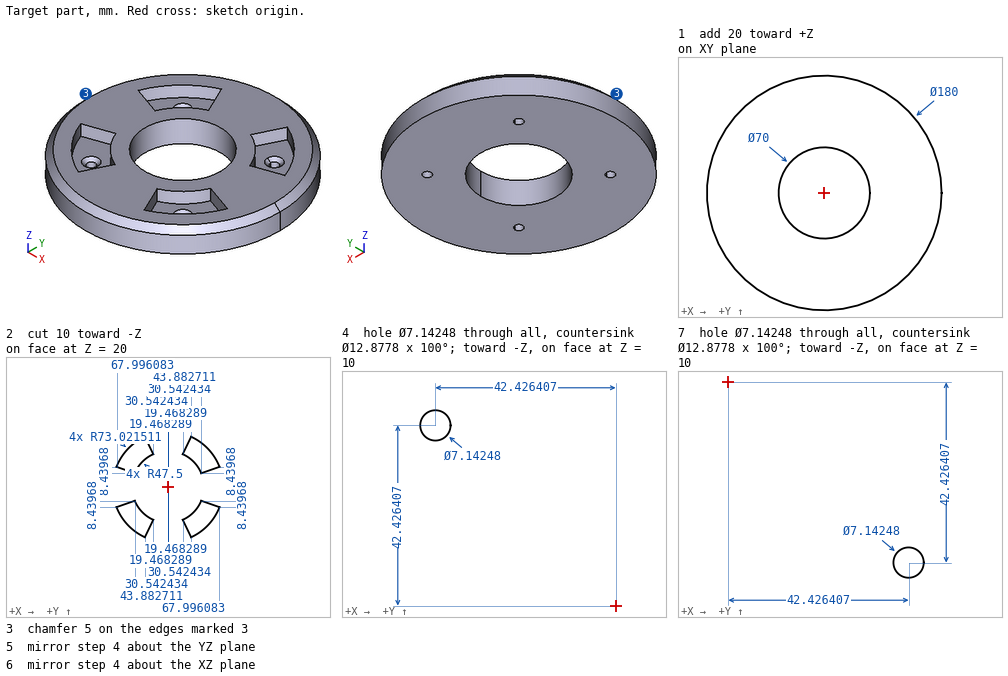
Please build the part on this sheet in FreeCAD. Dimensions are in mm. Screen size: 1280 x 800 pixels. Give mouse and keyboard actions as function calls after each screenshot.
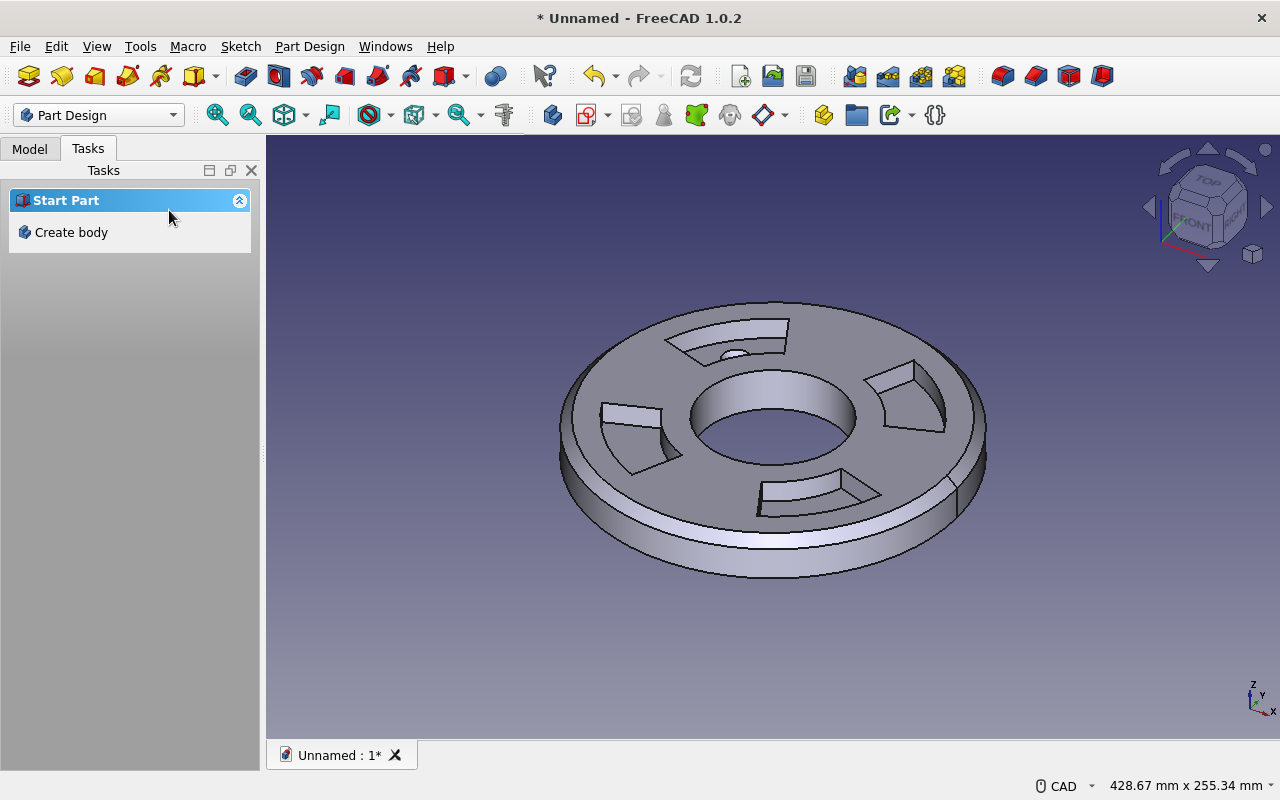
click(30, 148)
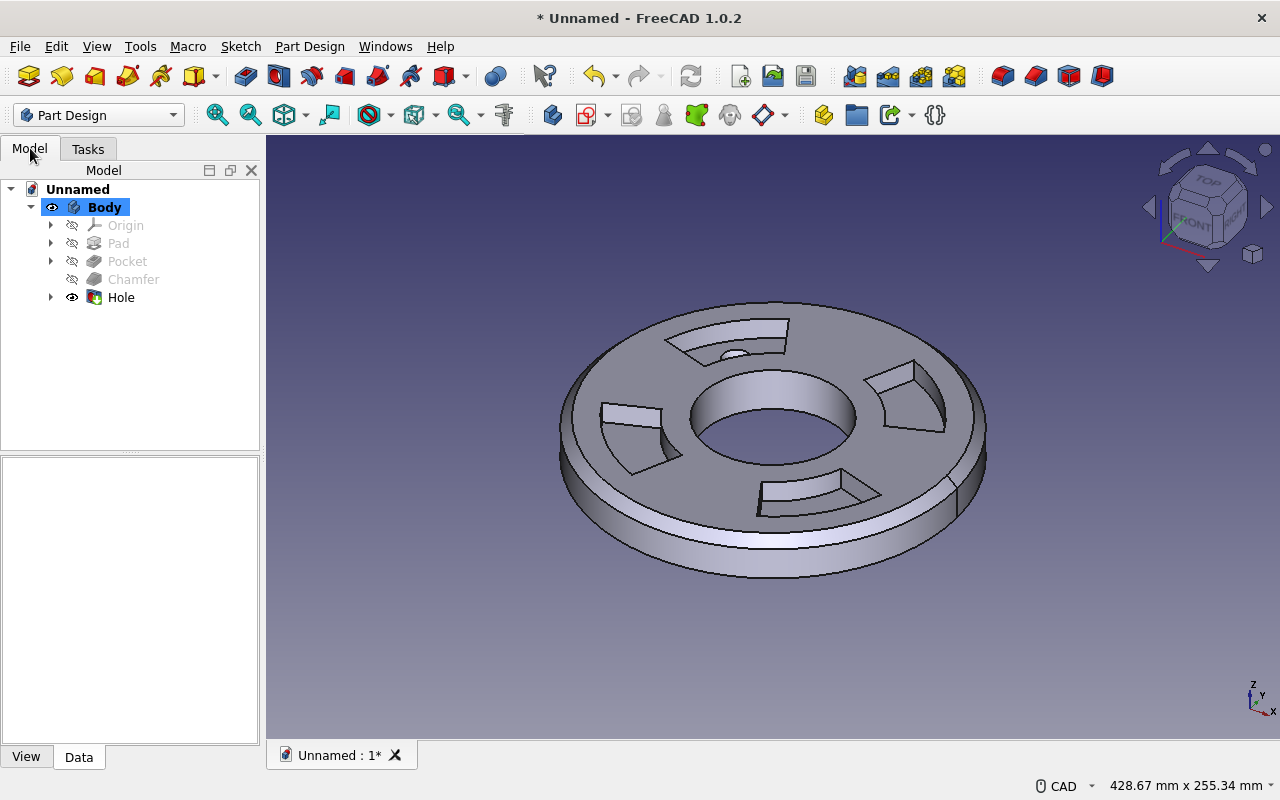
click(117, 297)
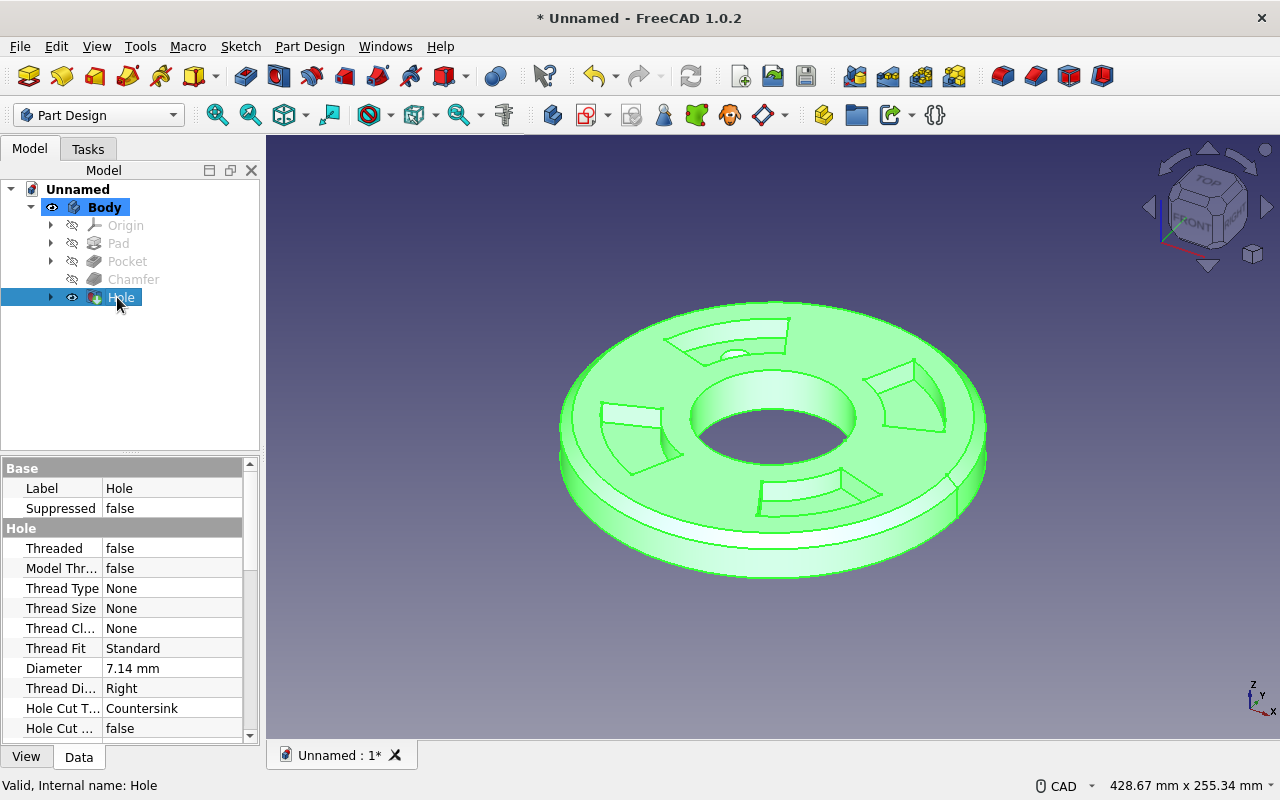
click(855, 76)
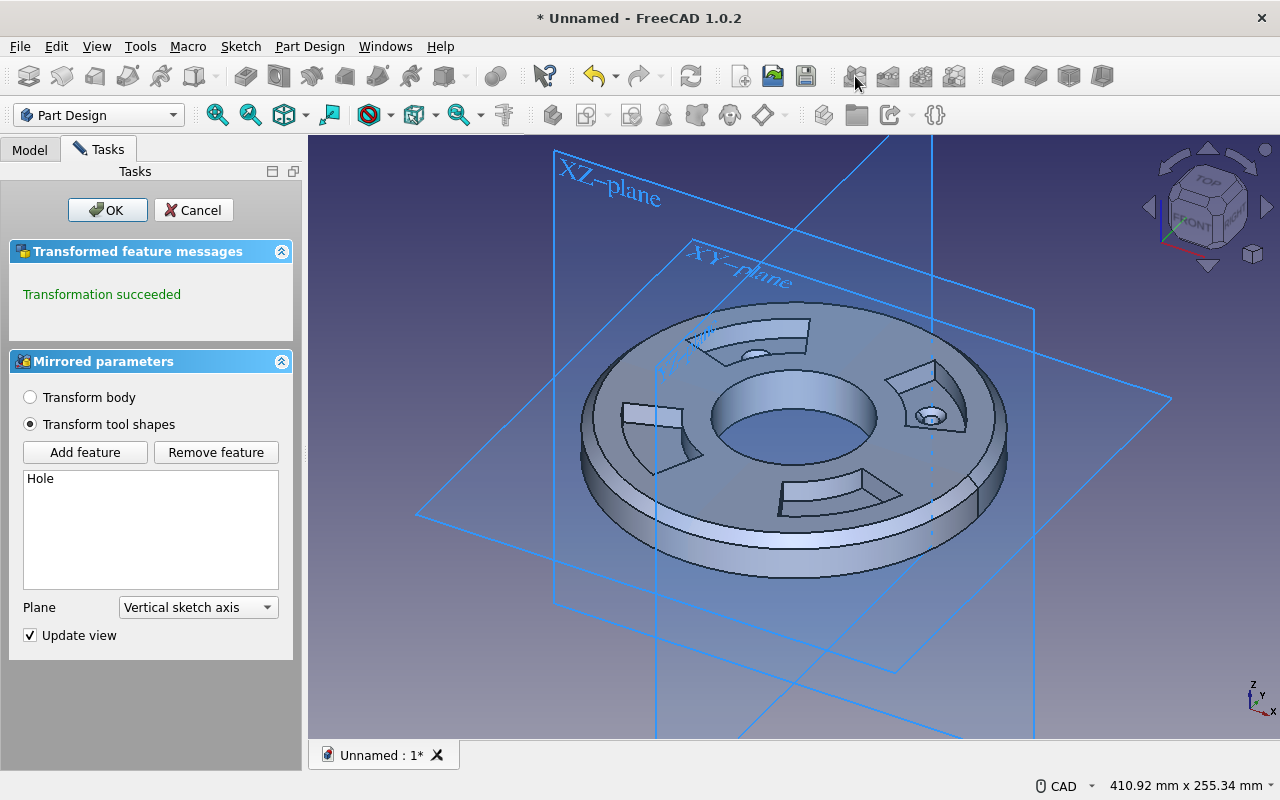
click(199, 608)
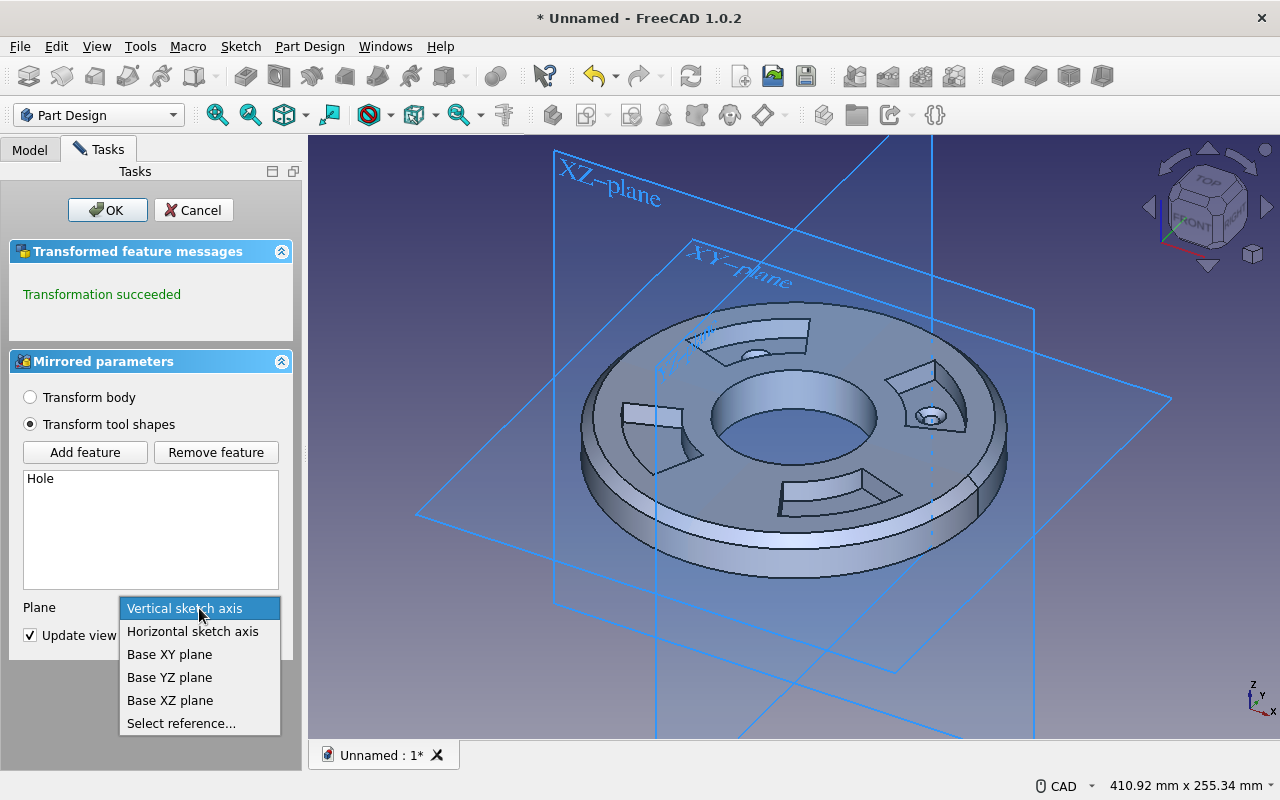
click(198, 678)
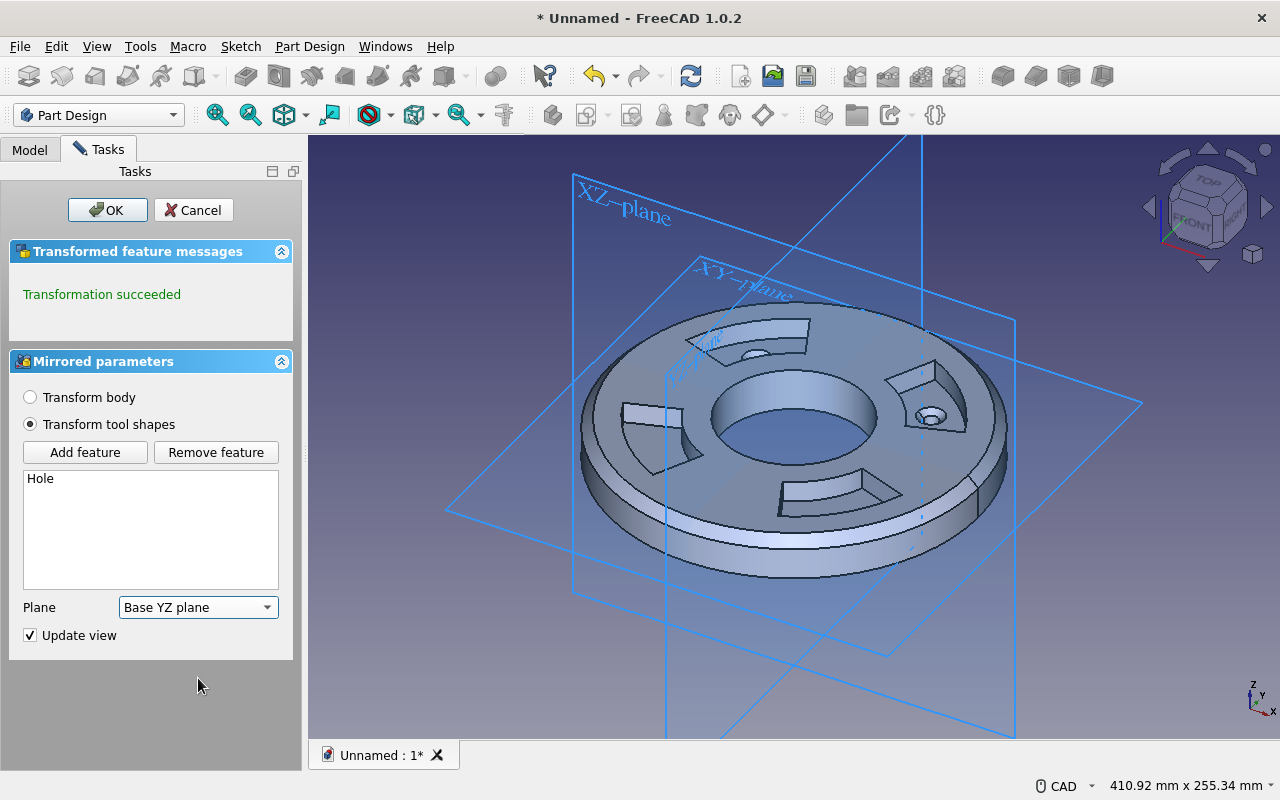
click(108, 210)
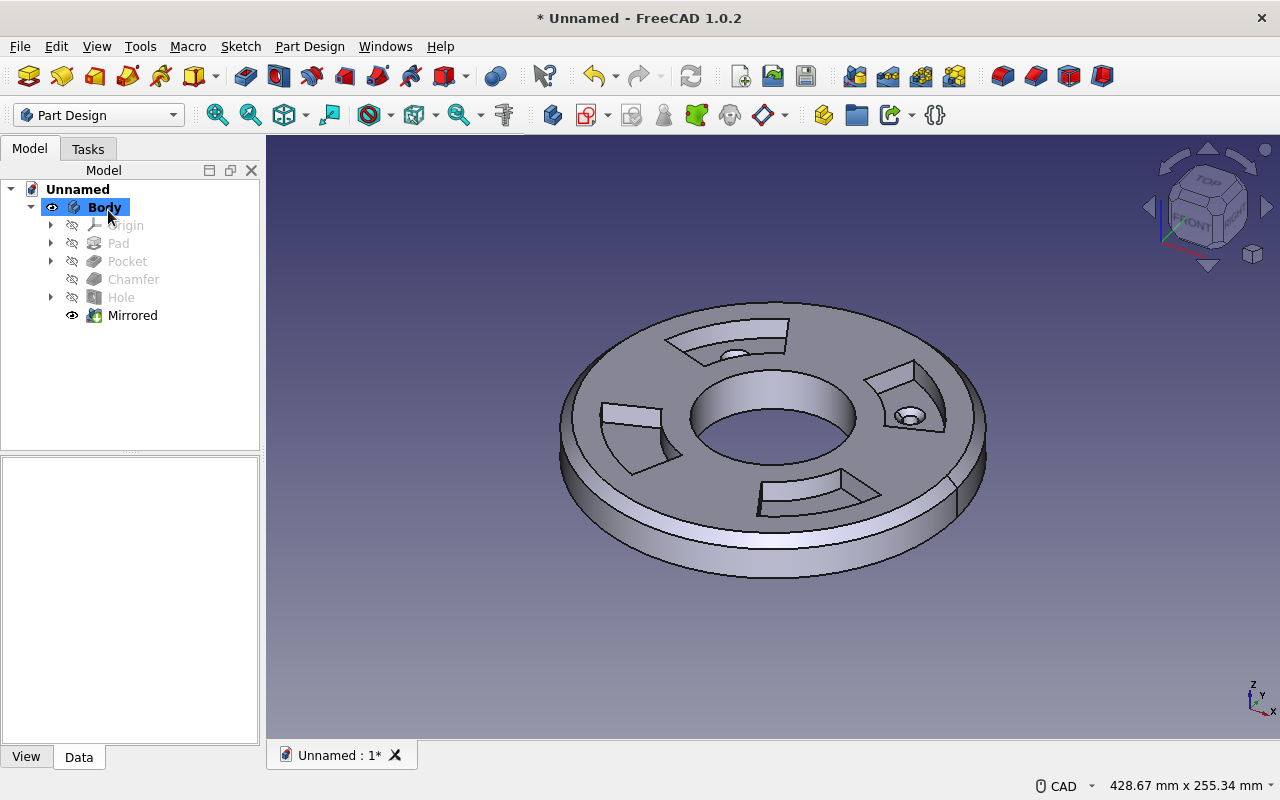
click(117, 297)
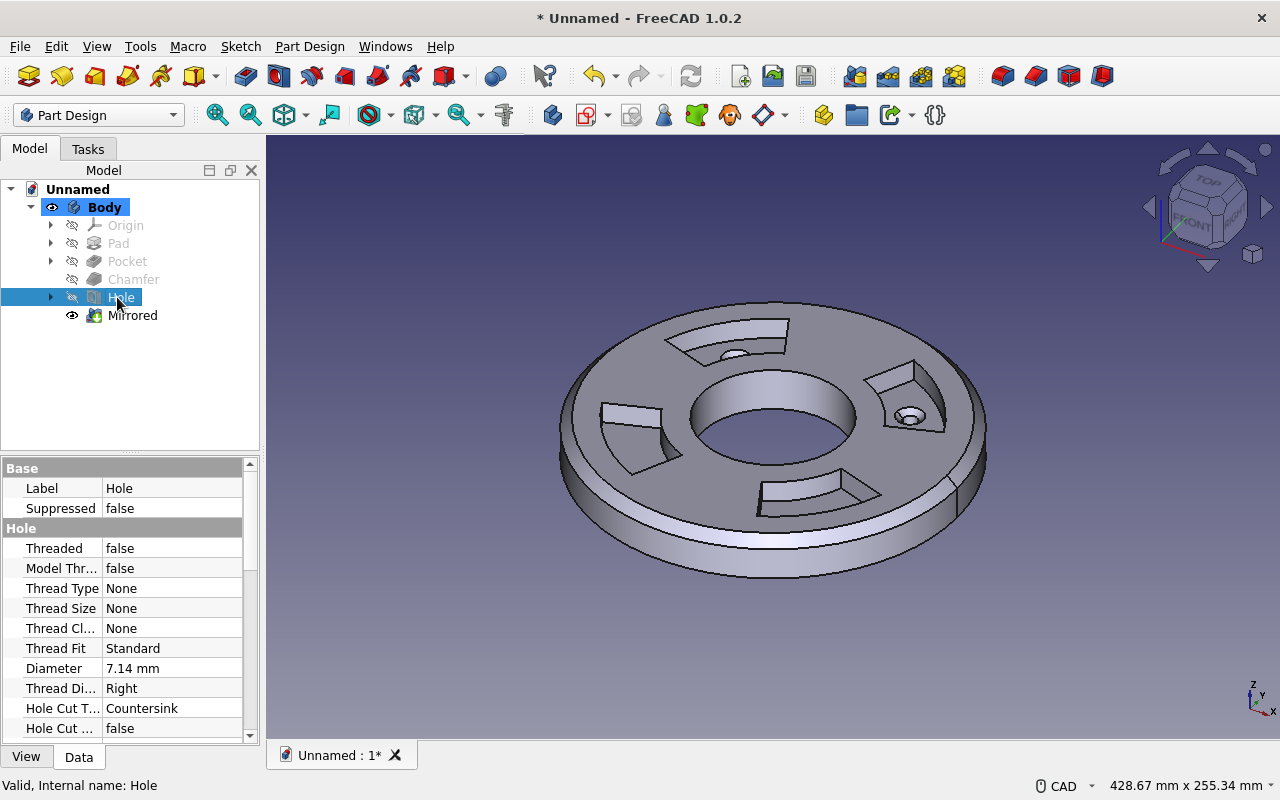
click(855, 76)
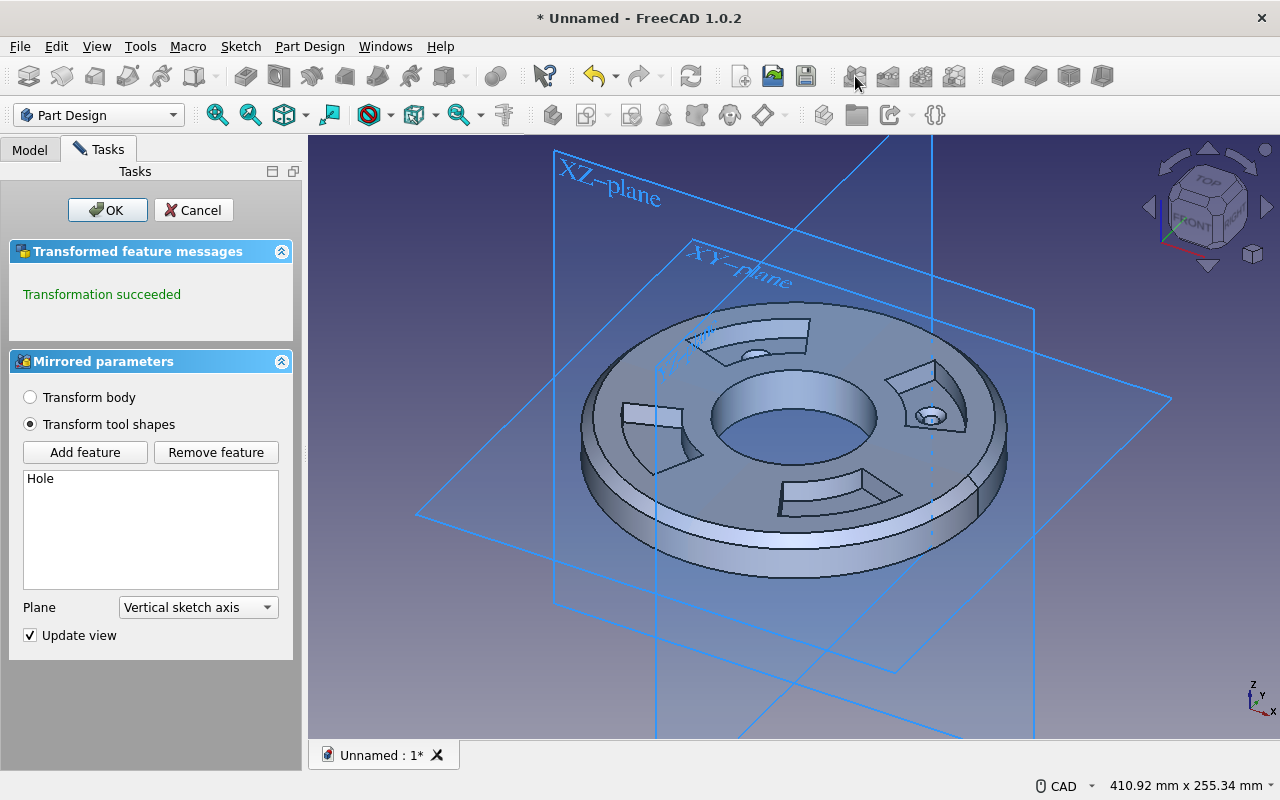
click(199, 608)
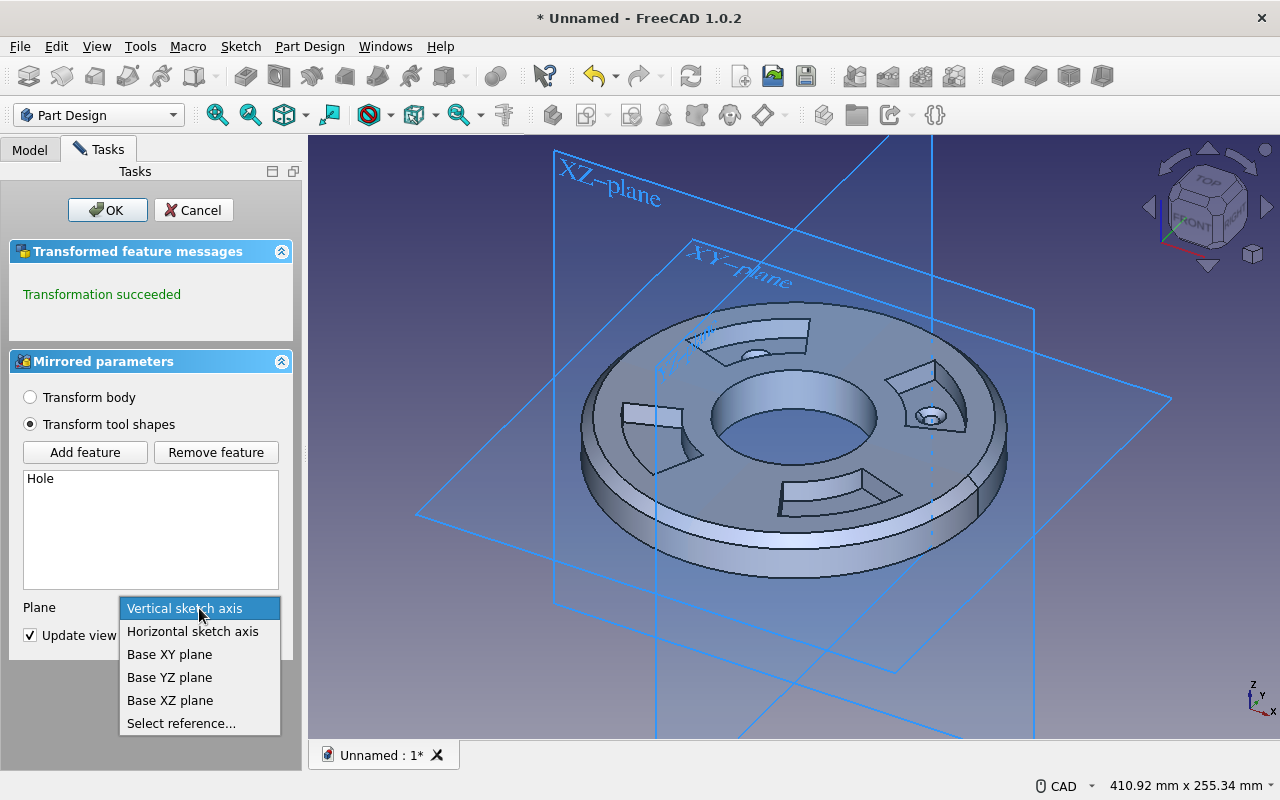
click(198, 700)